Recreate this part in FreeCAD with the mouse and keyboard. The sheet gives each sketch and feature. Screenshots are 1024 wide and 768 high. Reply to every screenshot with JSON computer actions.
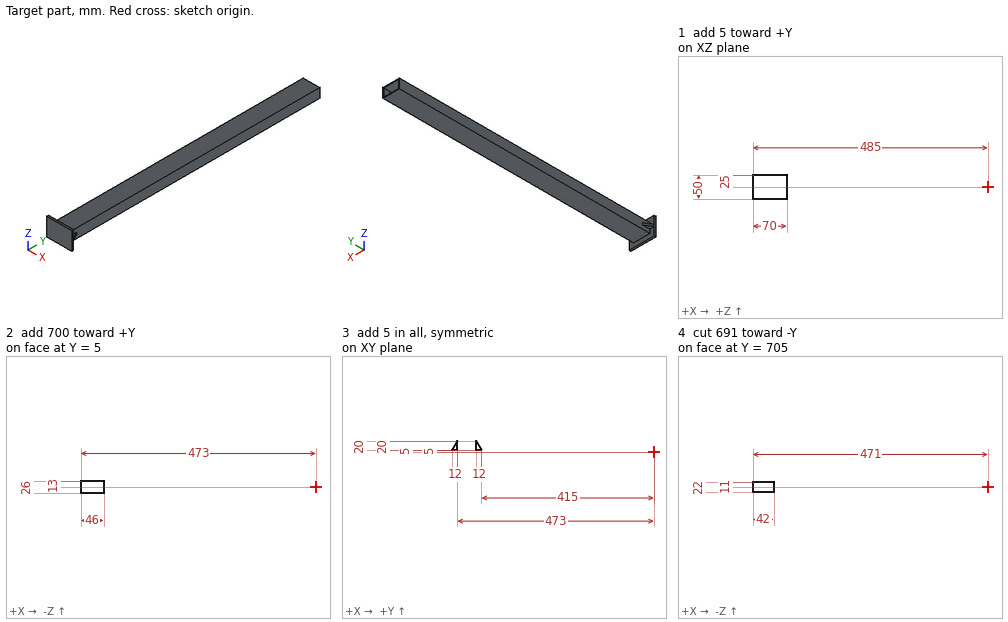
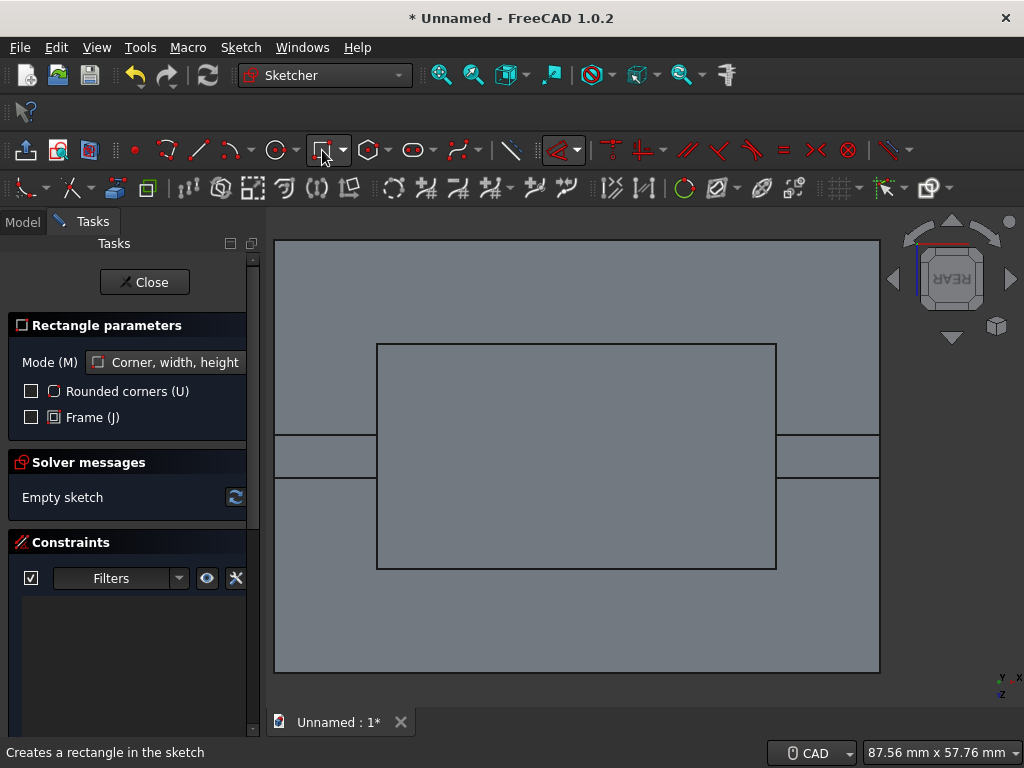
{"action": "left_click", "coordinate": [395, 362]}
{"action": "left_click", "coordinate": [758, 552]}
{"action": "key", "text": "Escape"}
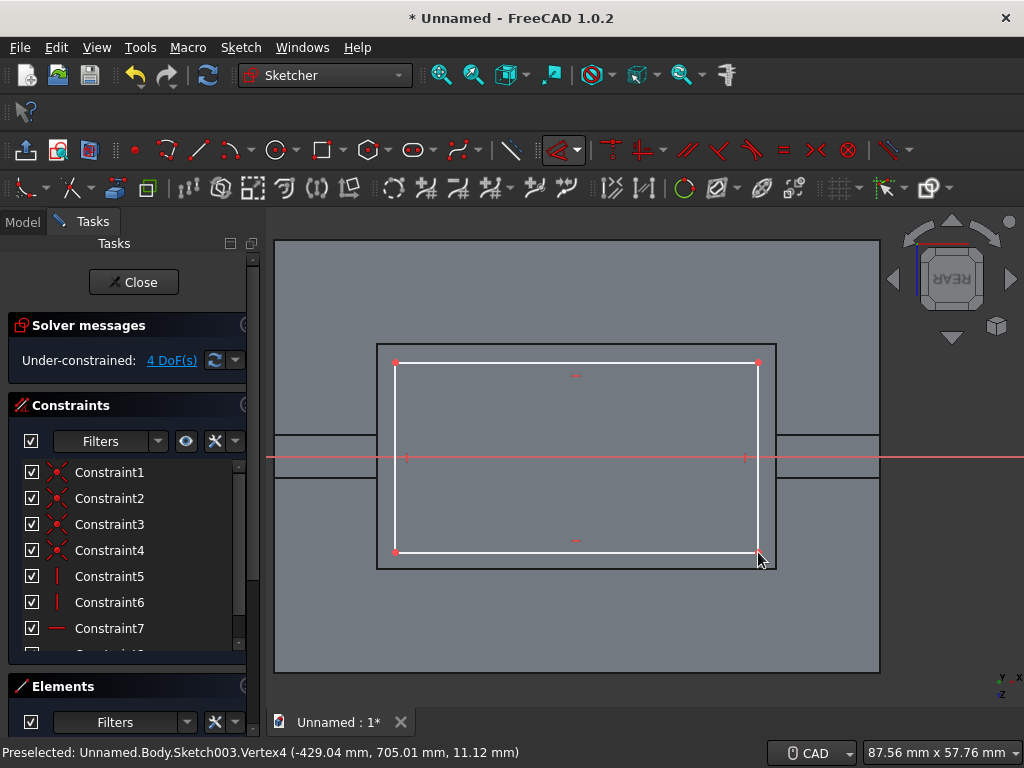
{"action": "left_click", "coordinate": [395, 420]}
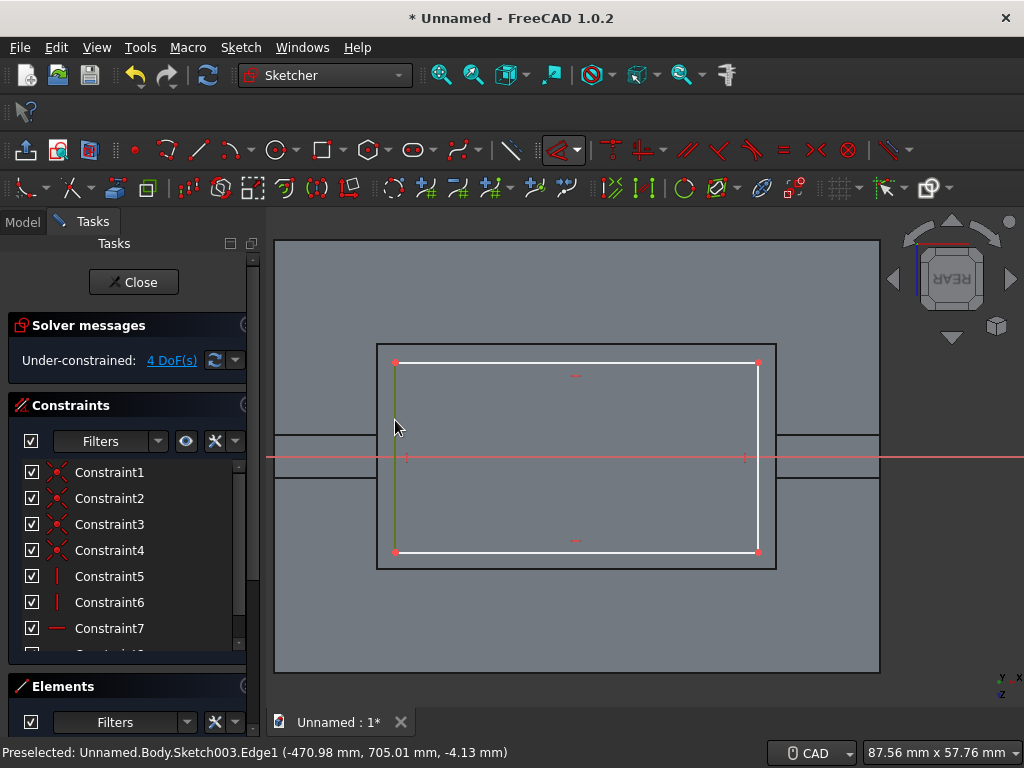
{"action": "left_click", "coordinate": [580, 150]}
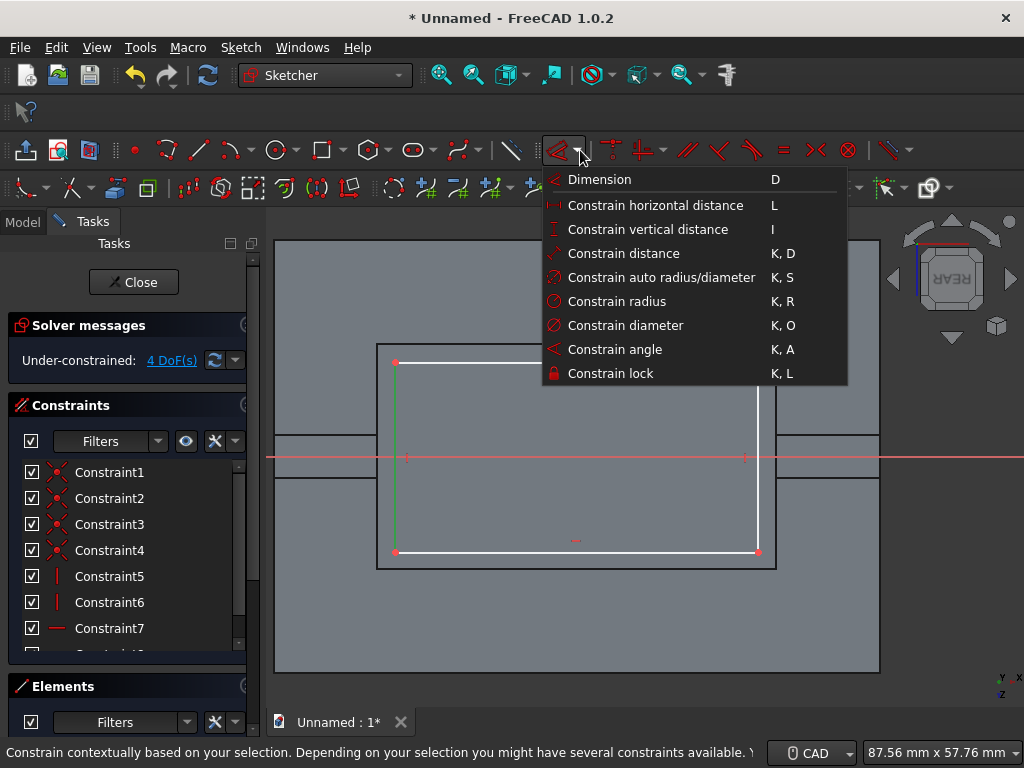
{"action": "left_click", "coordinate": [695, 229]}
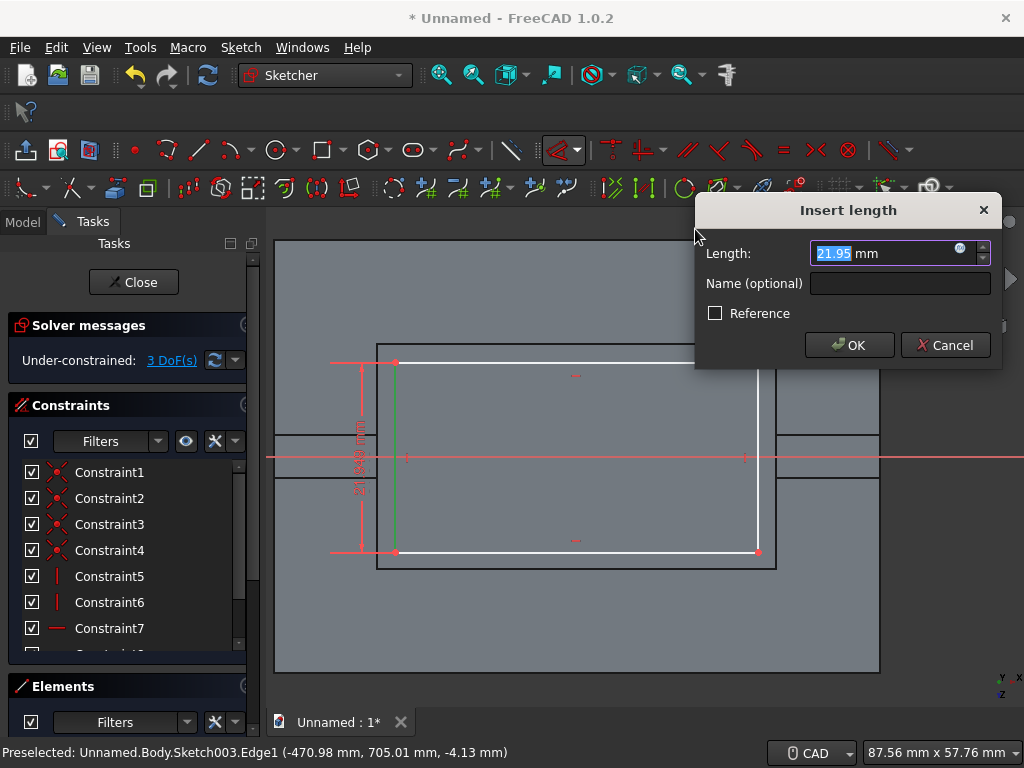
{"action": "type", "text": "22"}
{"action": "key", "text": "Return"}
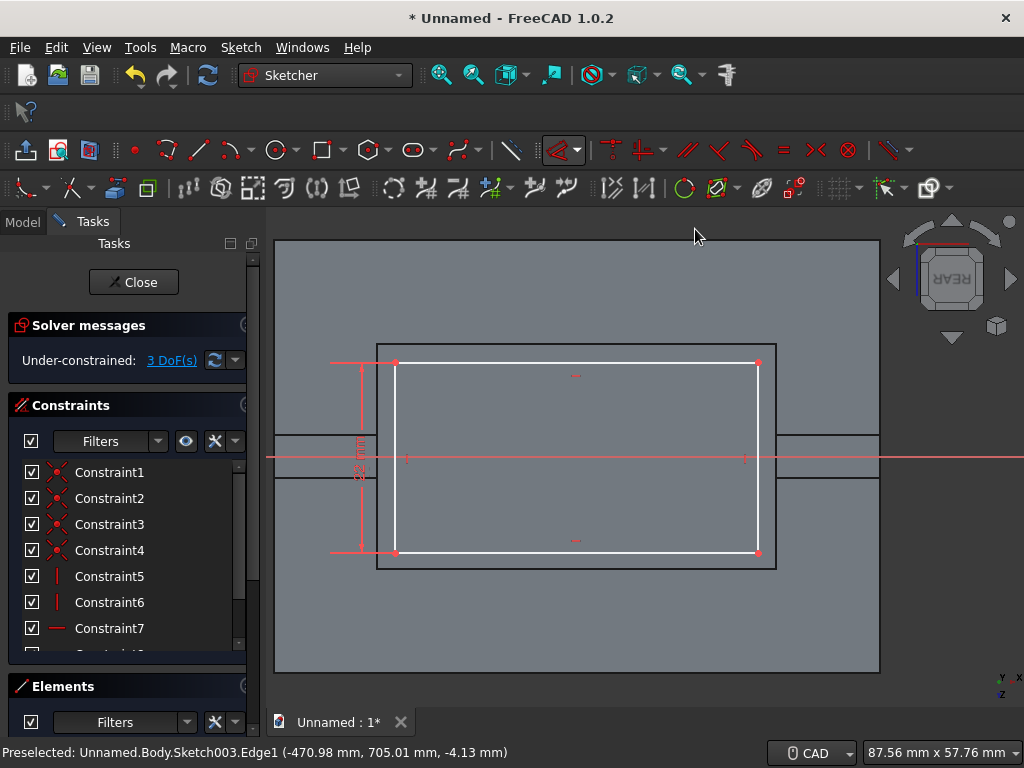
{"action": "left_click", "coordinate": [504, 553]}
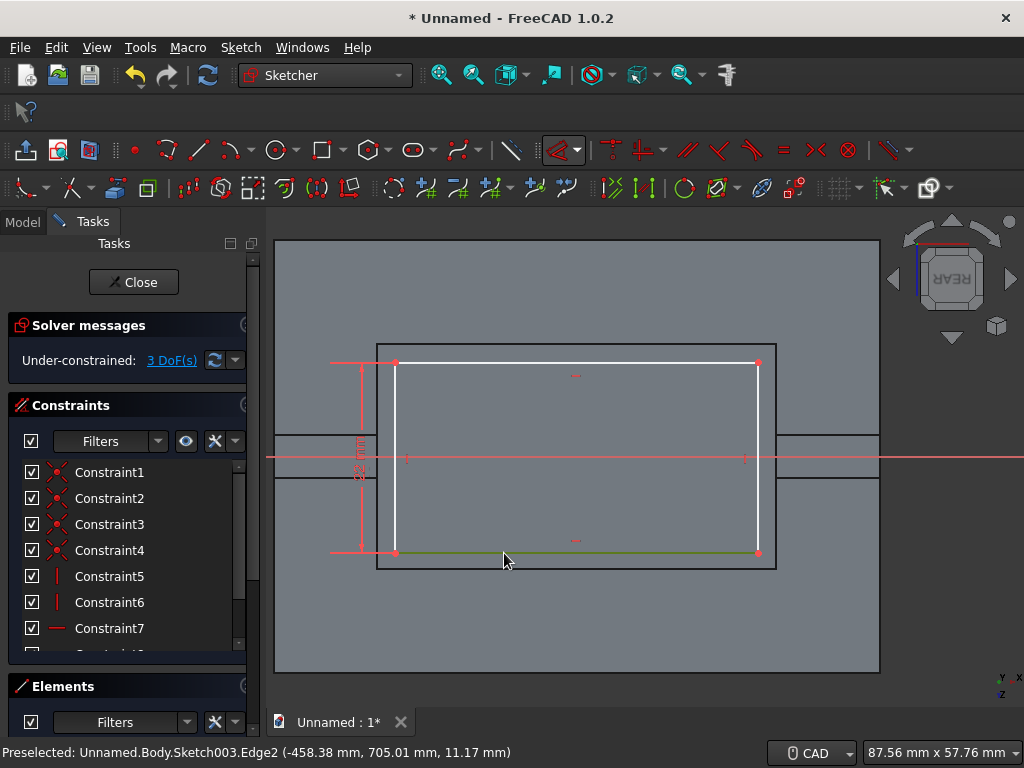
{"action": "left_click", "coordinate": [580, 150]}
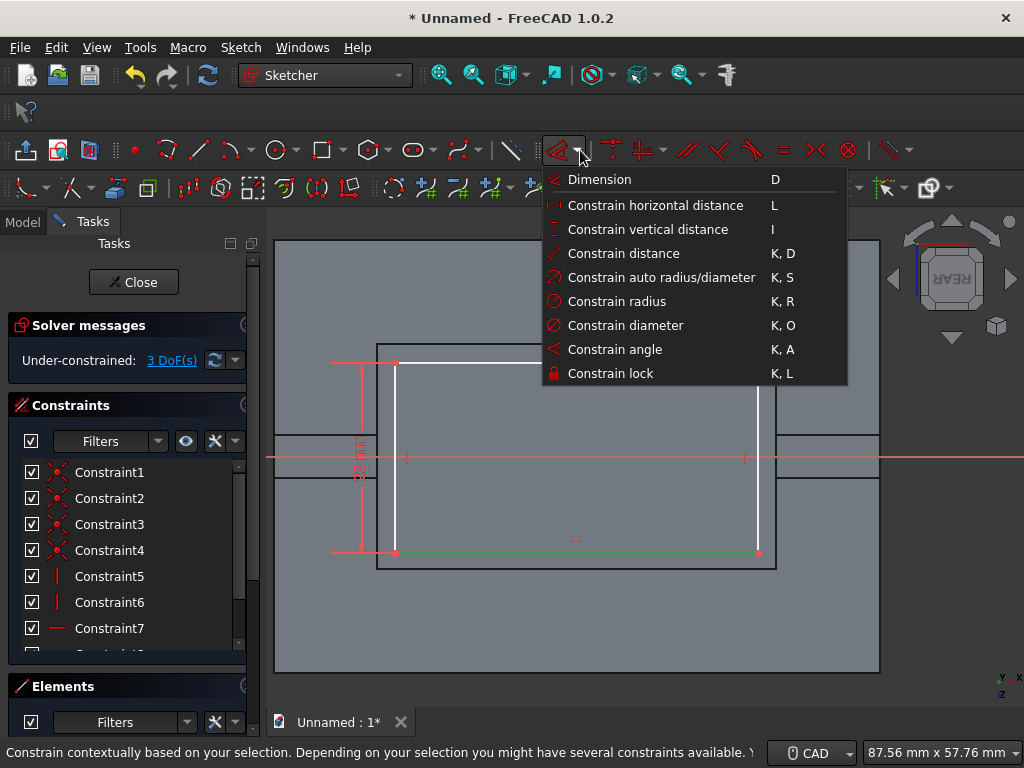
{"action": "left_click", "coordinate": [695, 205]}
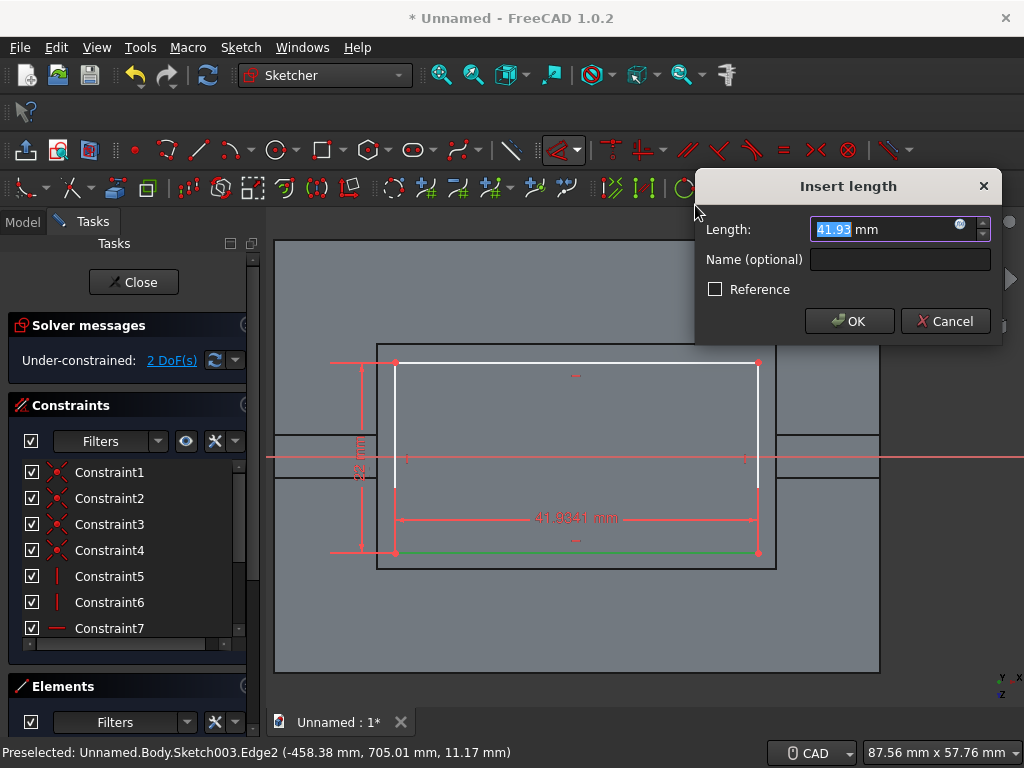
{"action": "type", "text": "42"}
{"action": "key", "text": "Return"}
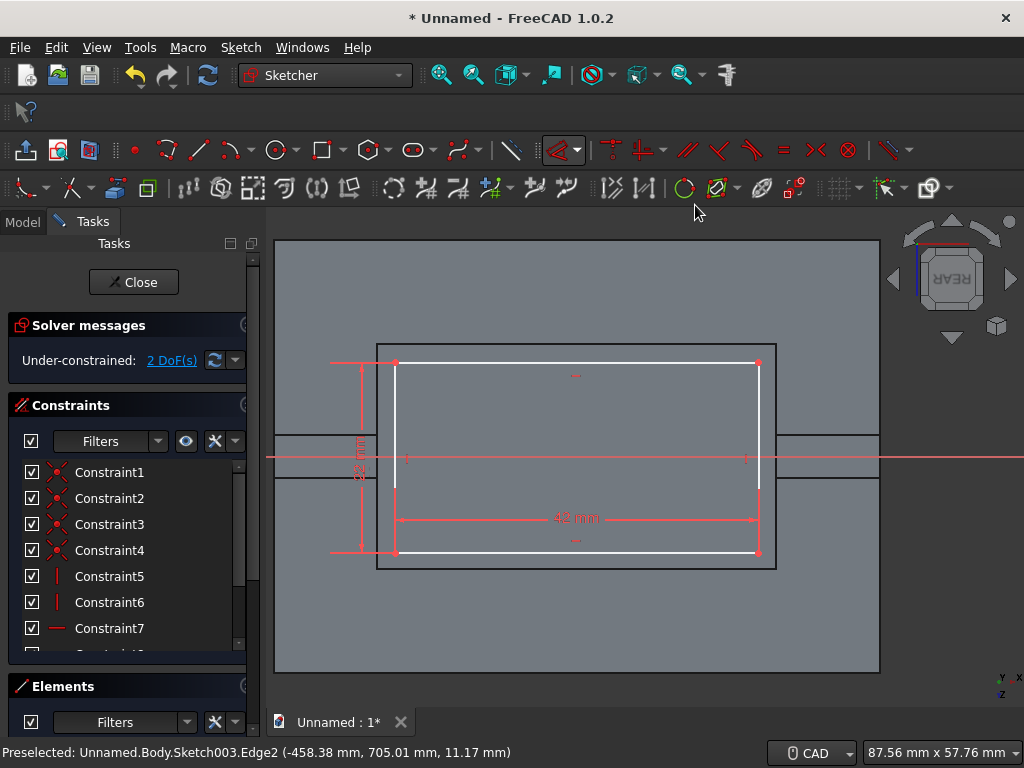
{"action": "left_click", "coordinate": [395, 363]}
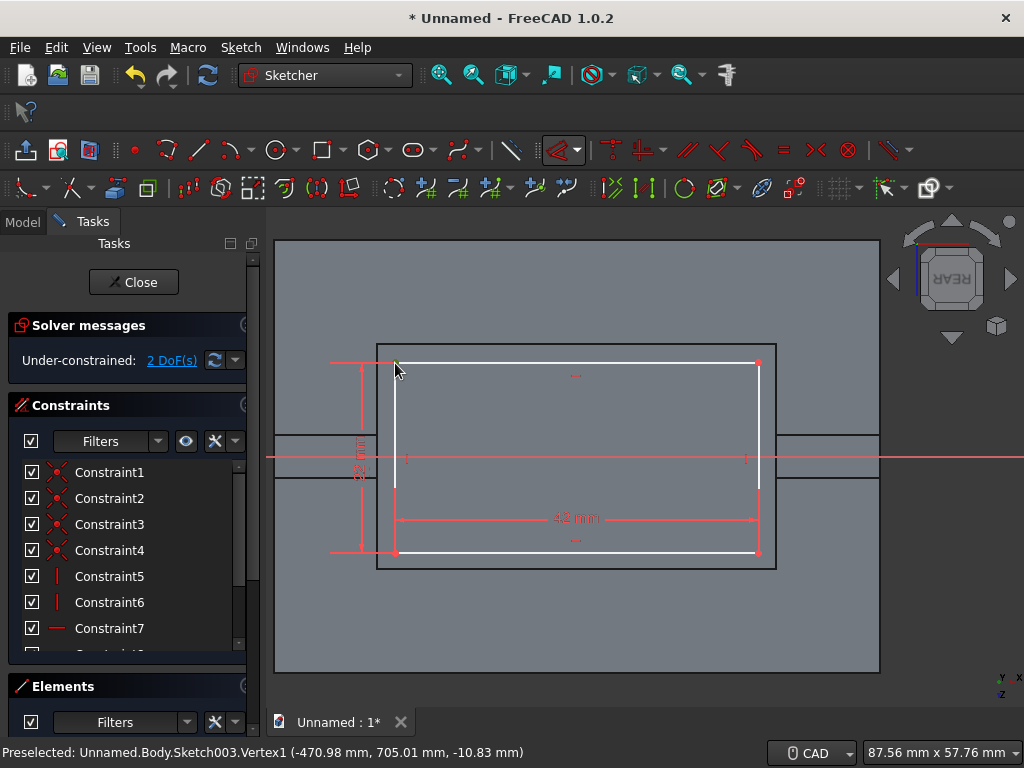
{"action": "key", "text": "i"}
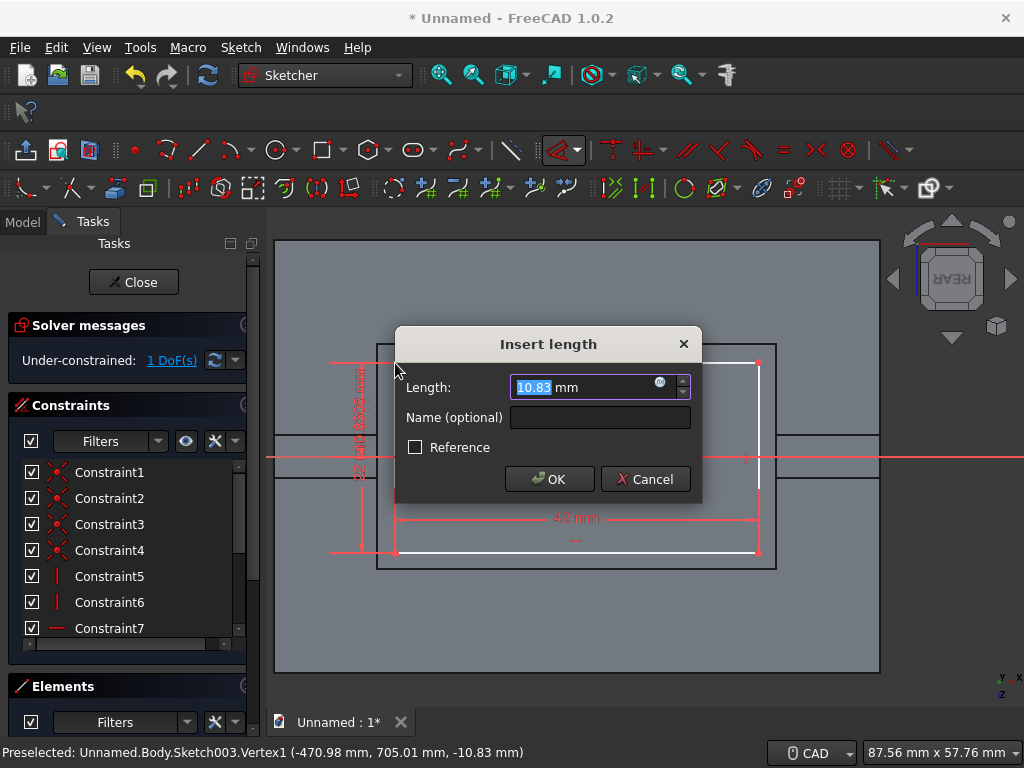
{"action": "type", "text": "11"}
{"action": "key", "text": "Return"}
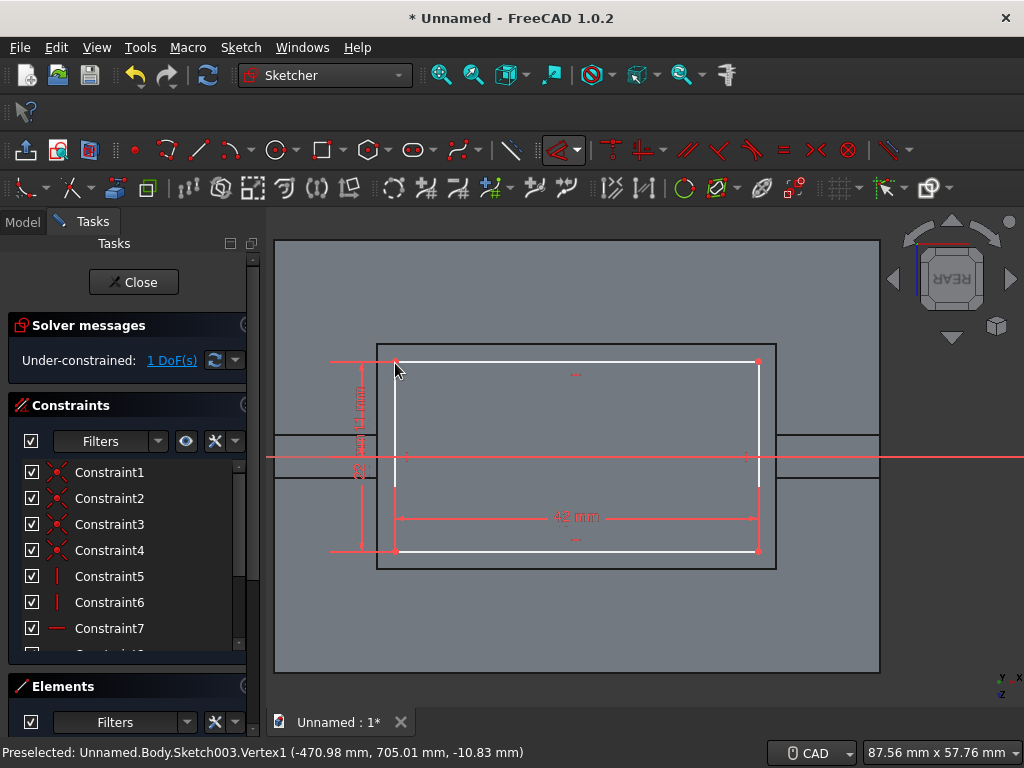
{"action": "left_click", "coordinate": [395, 362]}